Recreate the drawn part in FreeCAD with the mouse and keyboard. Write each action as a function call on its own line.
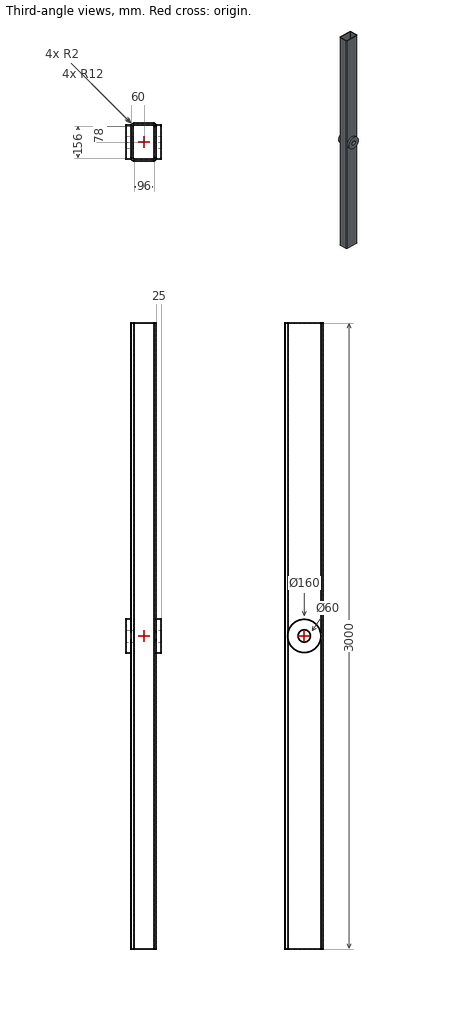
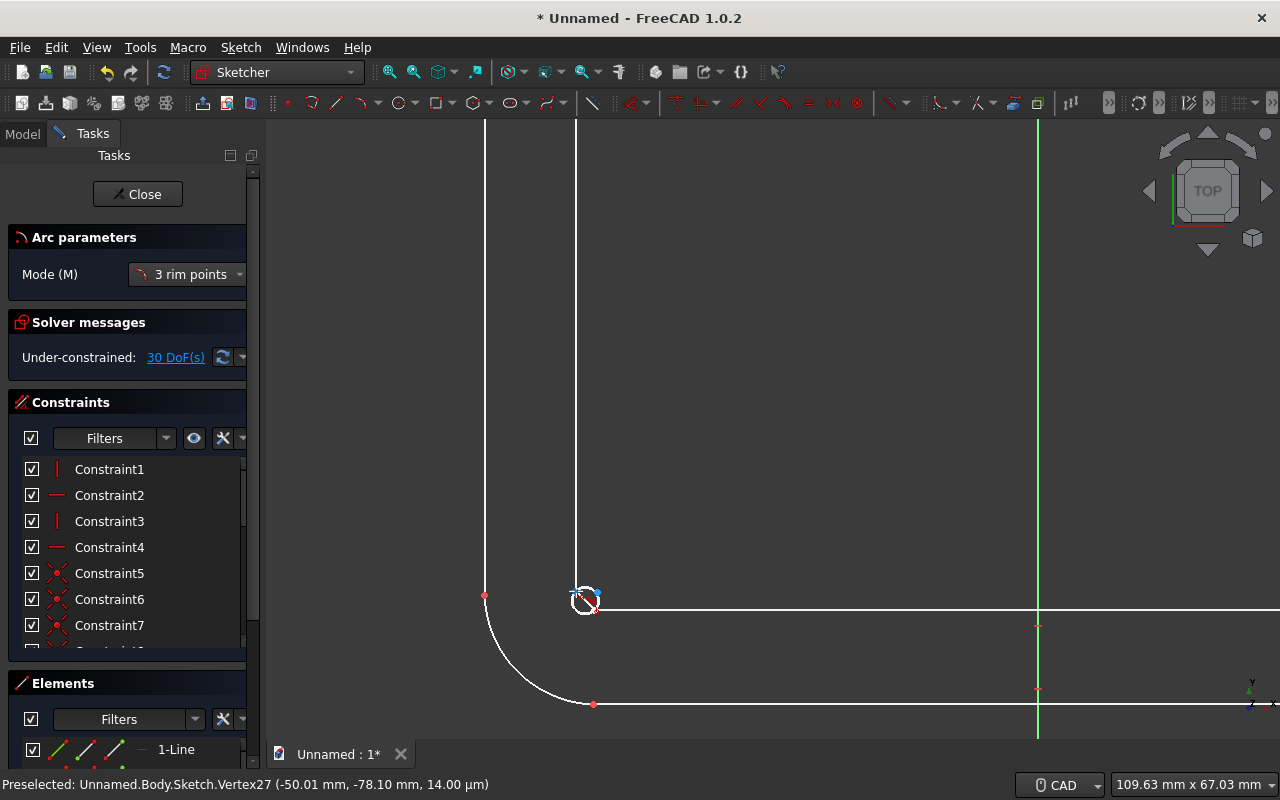
scroll(581, 603, up, 6)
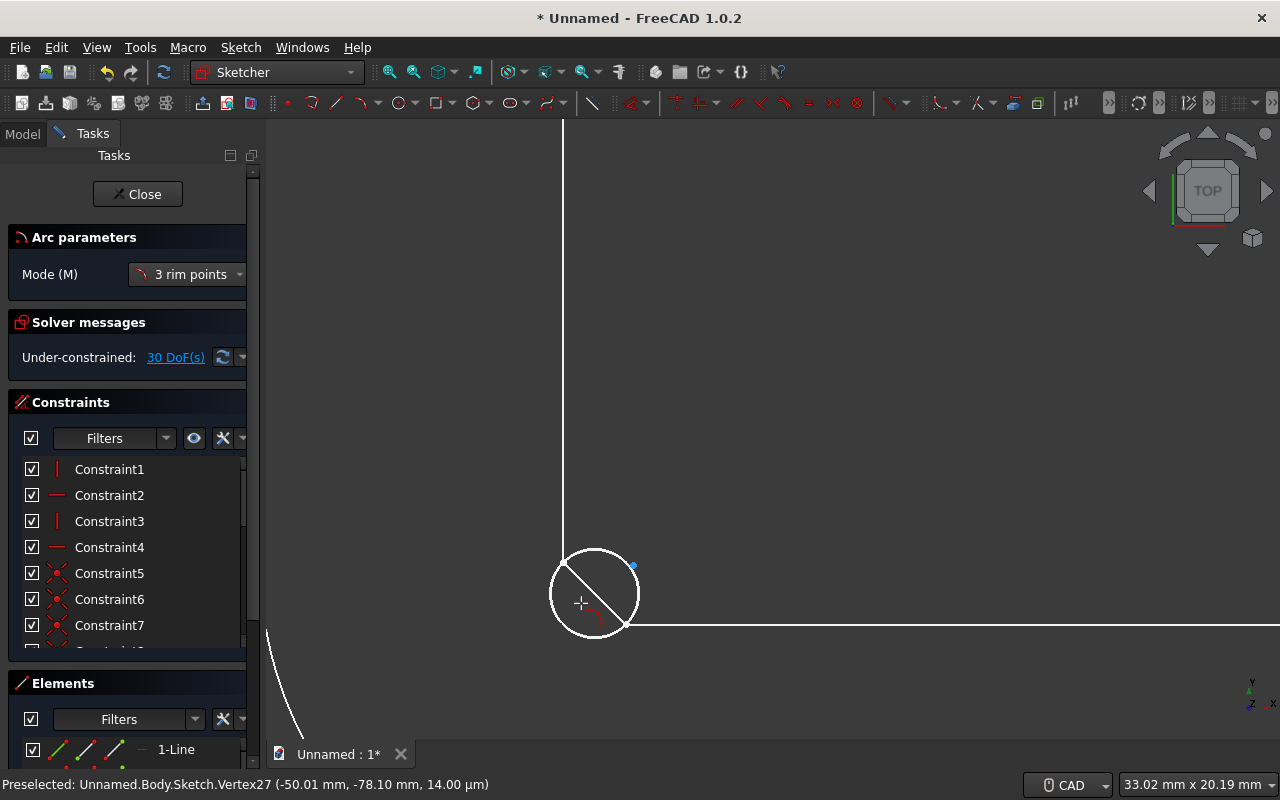
click(582, 603)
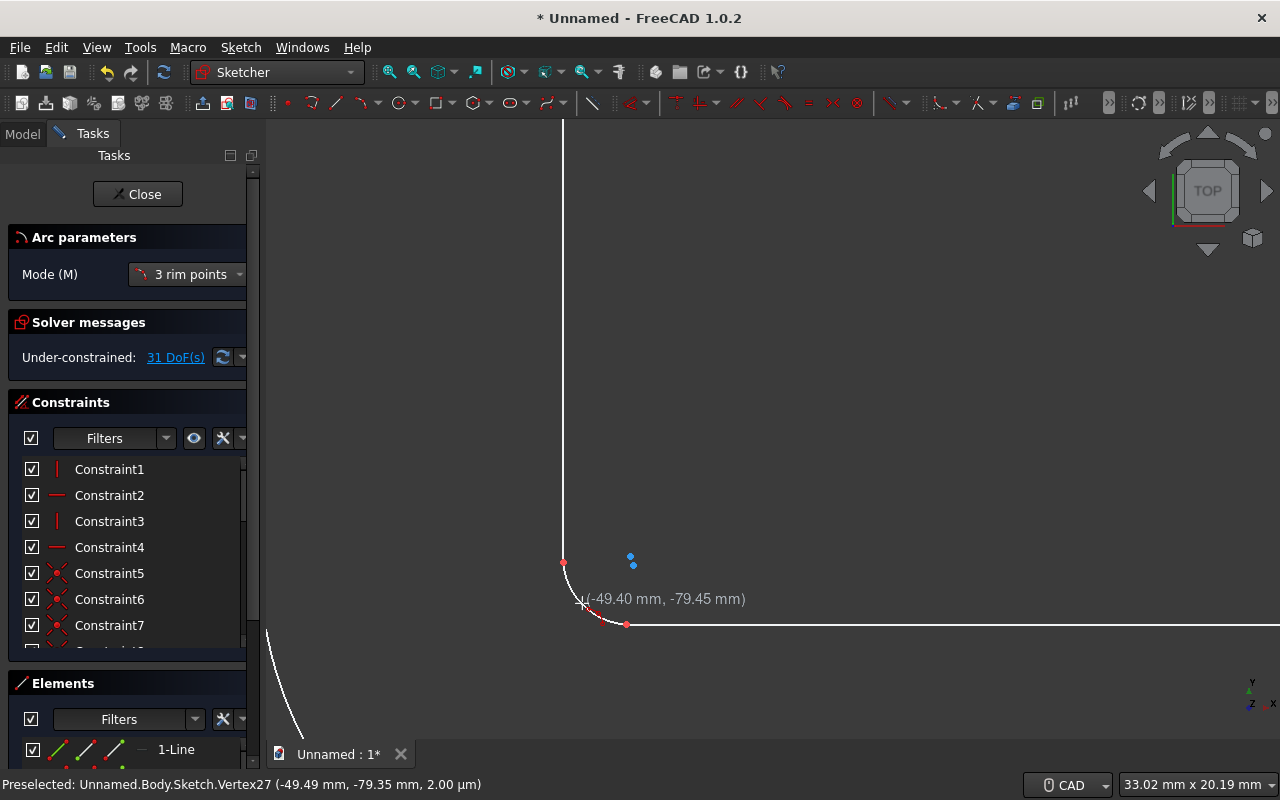
scroll(593, 611, down, 13)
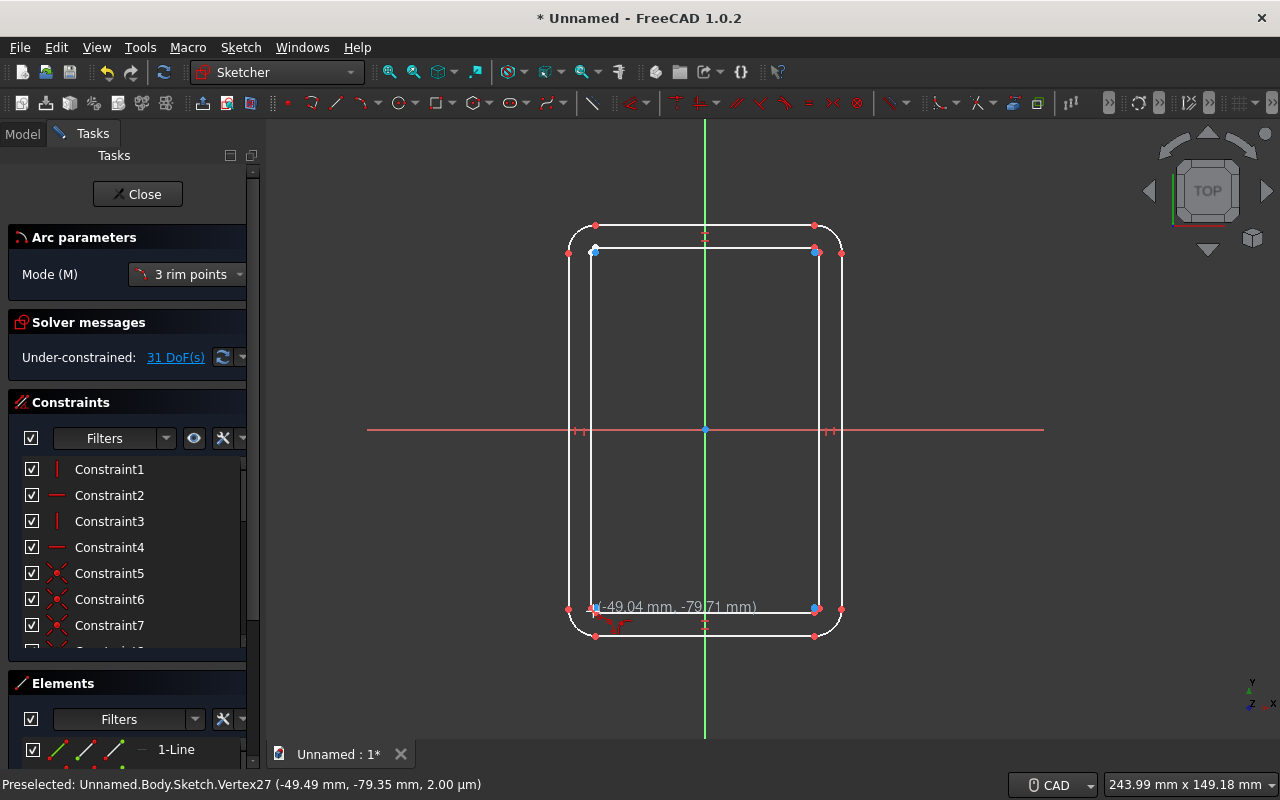
scroll(591, 252, up, 7)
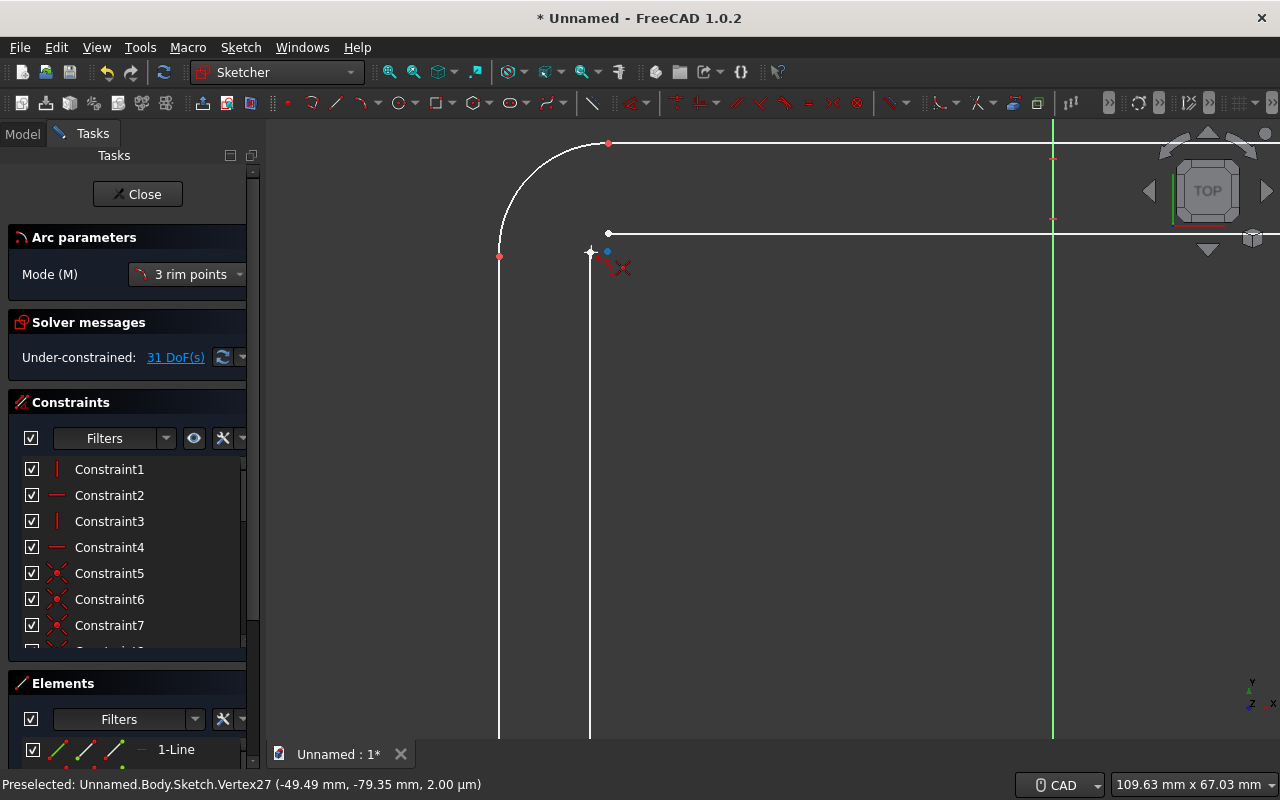
click(590, 252)
click(609, 234)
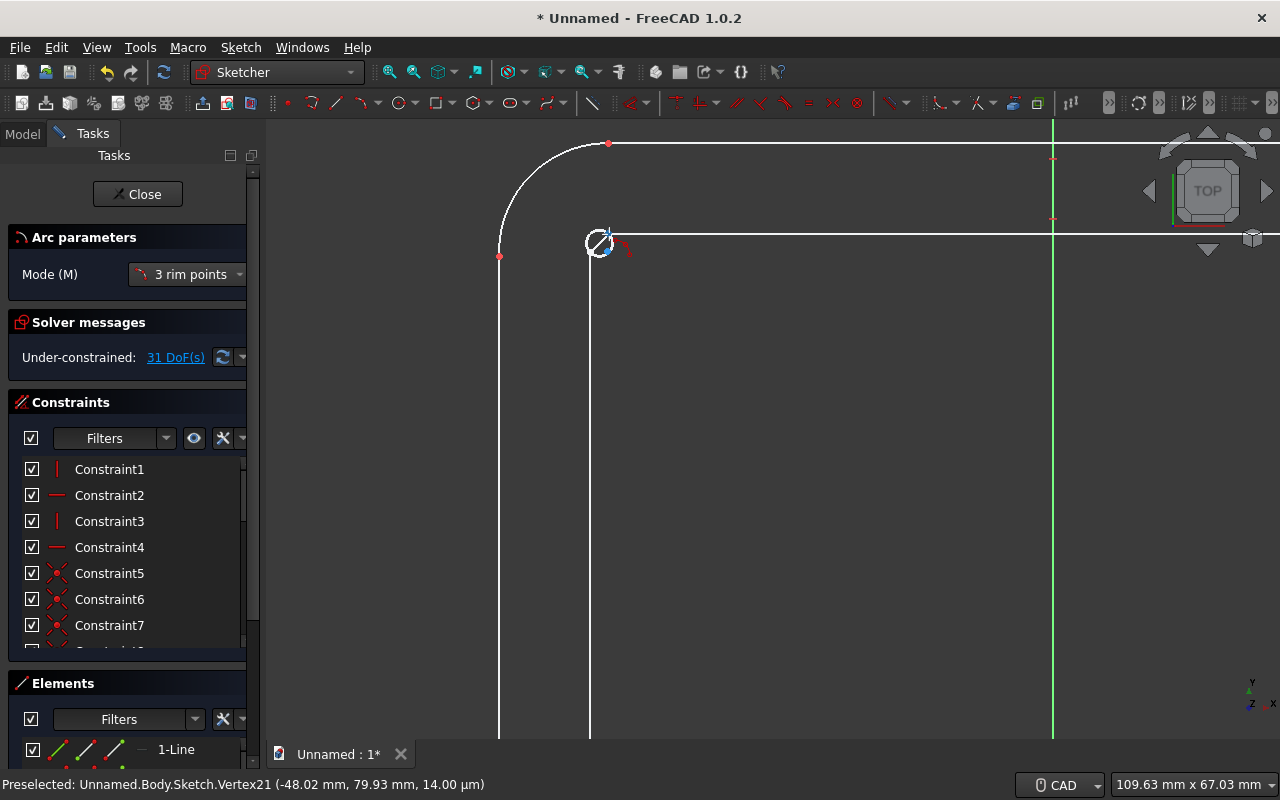
scroll(596, 239, up, 6)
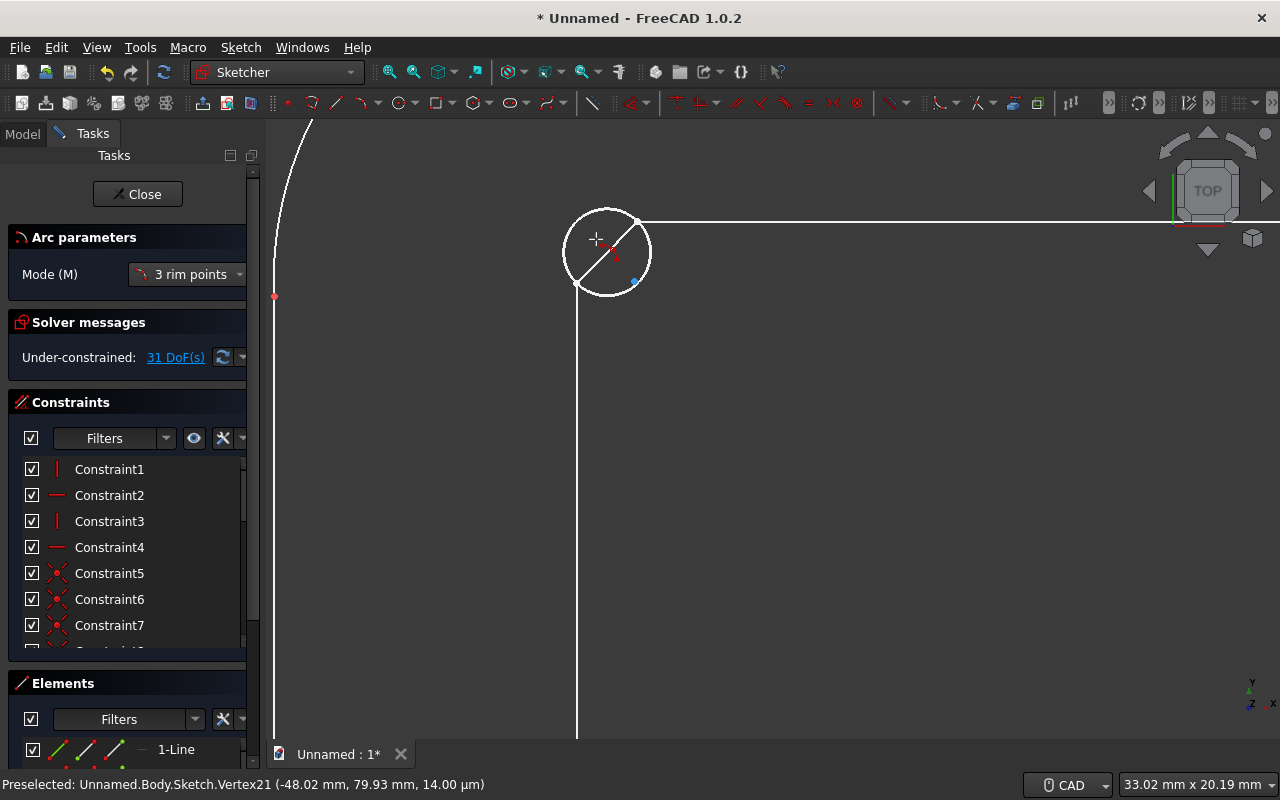
click(595, 237)
key(Escape)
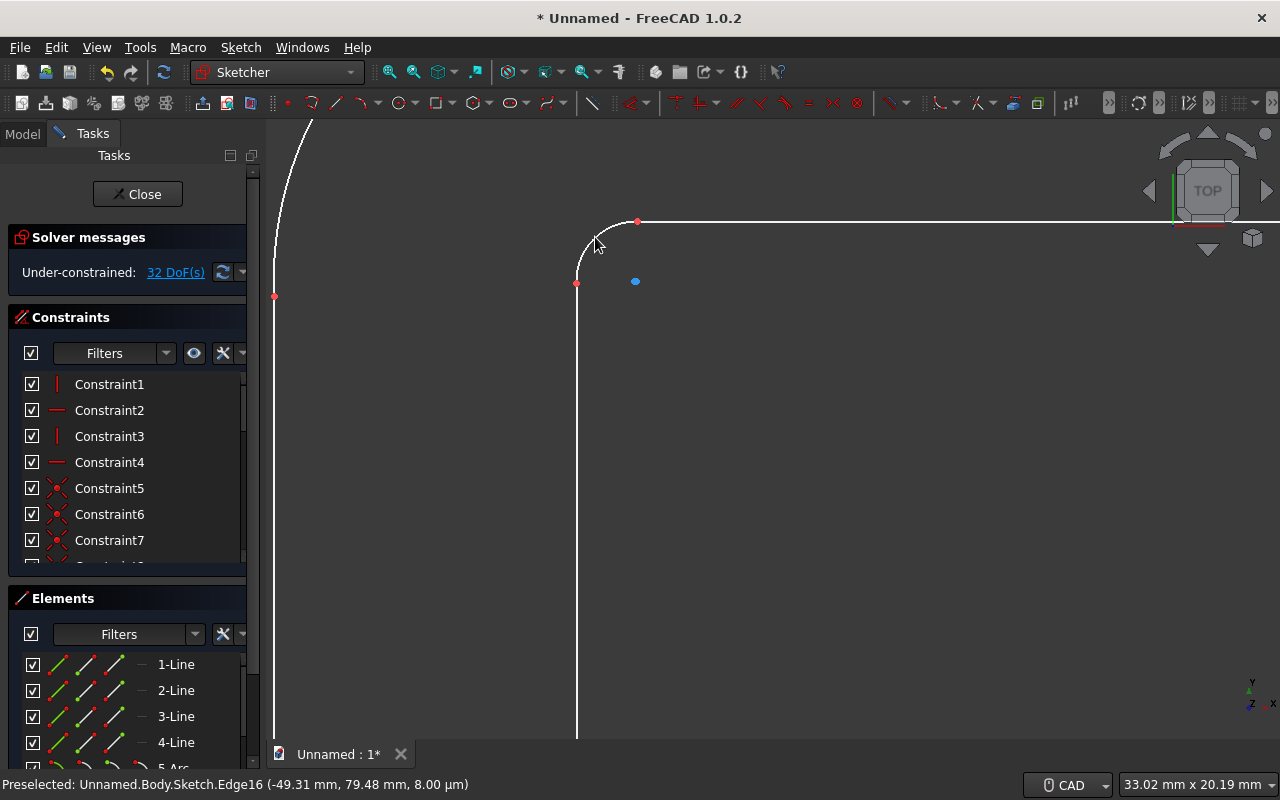
scroll(592, 249, down, 13)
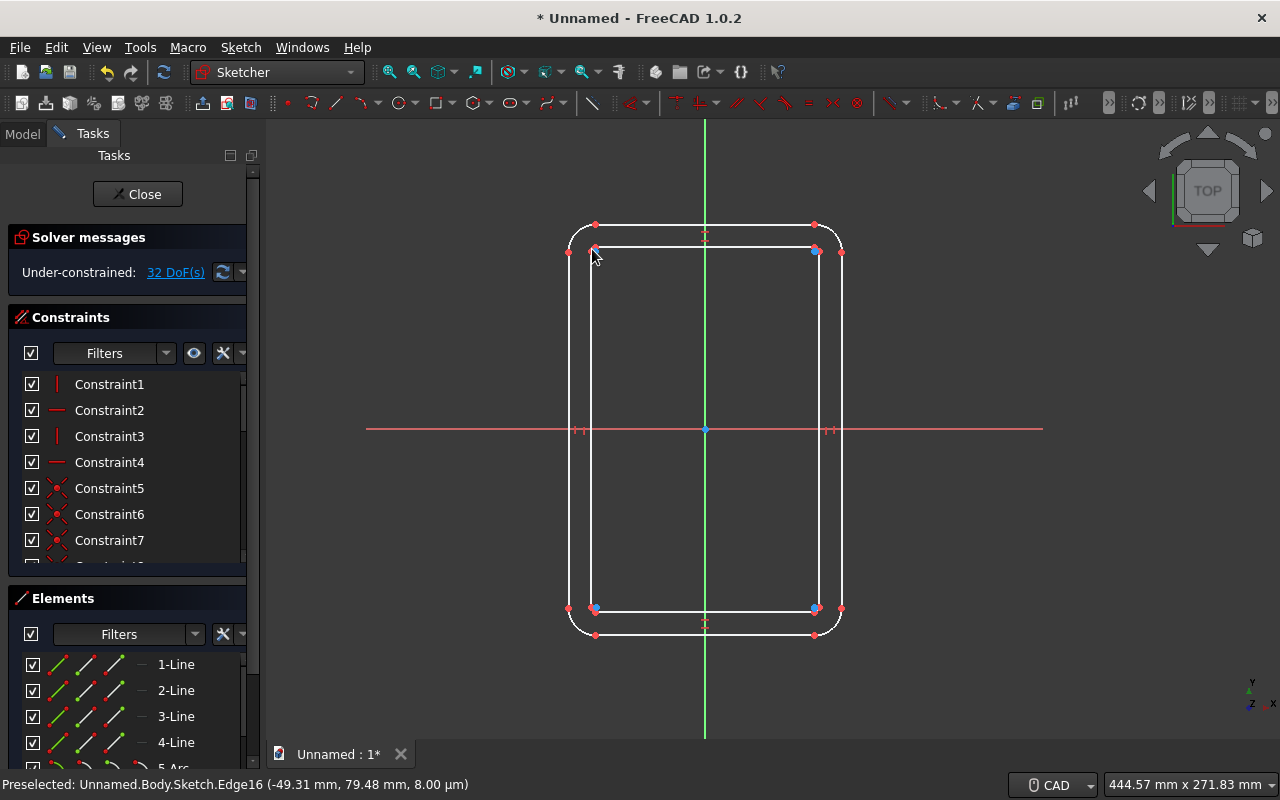
click(569, 359)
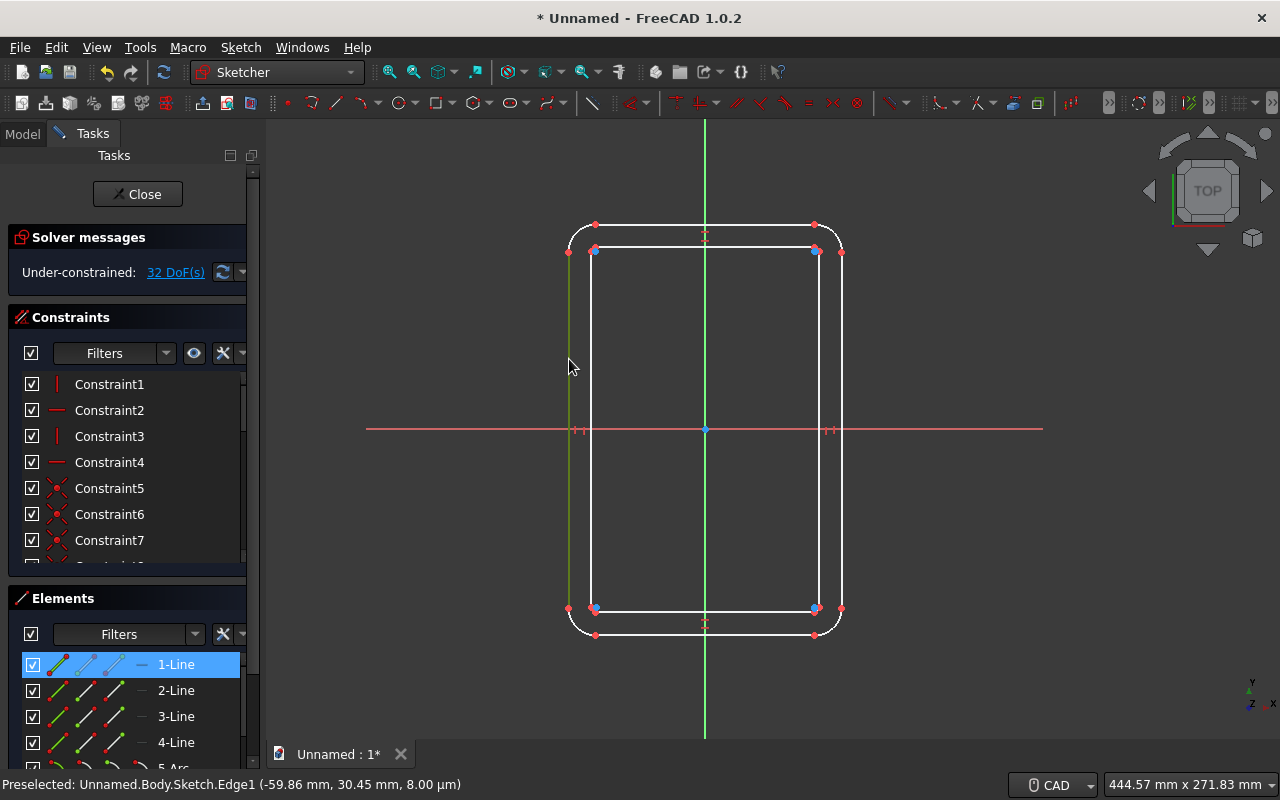
click(572, 621)